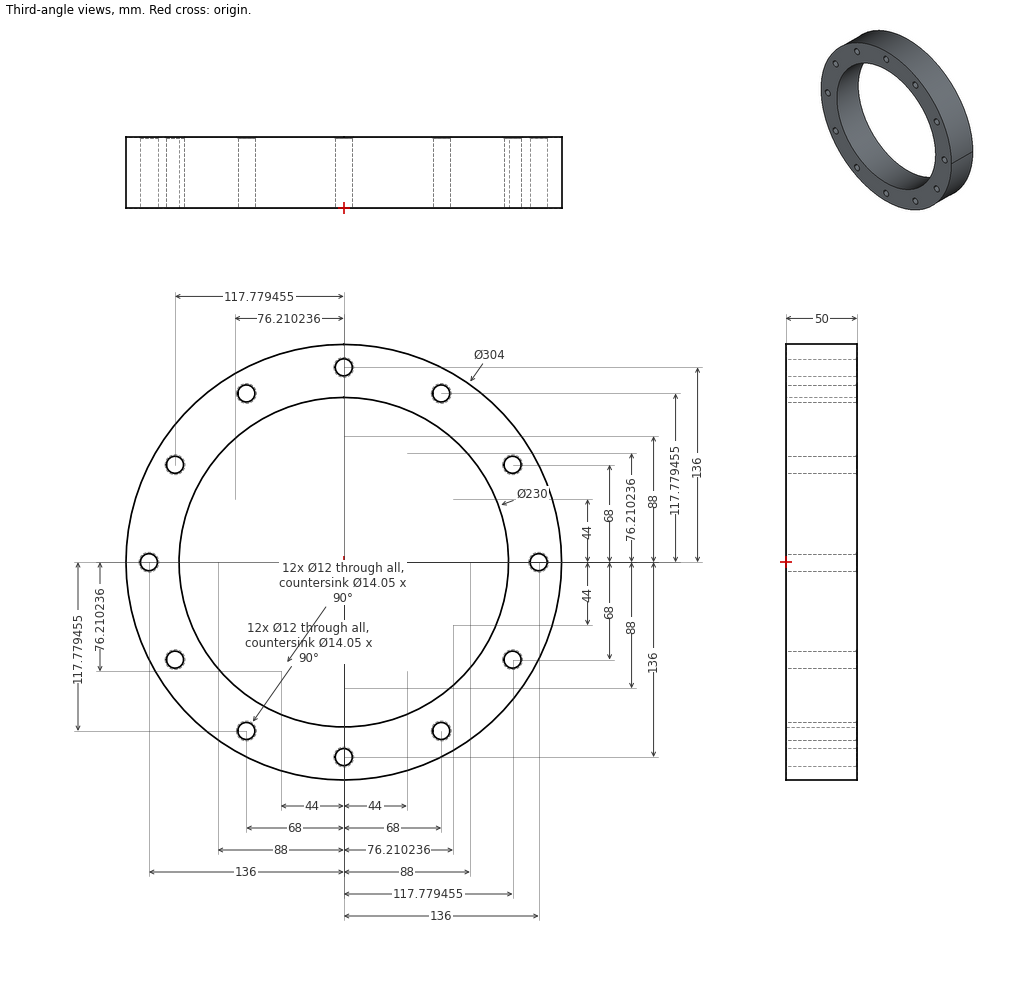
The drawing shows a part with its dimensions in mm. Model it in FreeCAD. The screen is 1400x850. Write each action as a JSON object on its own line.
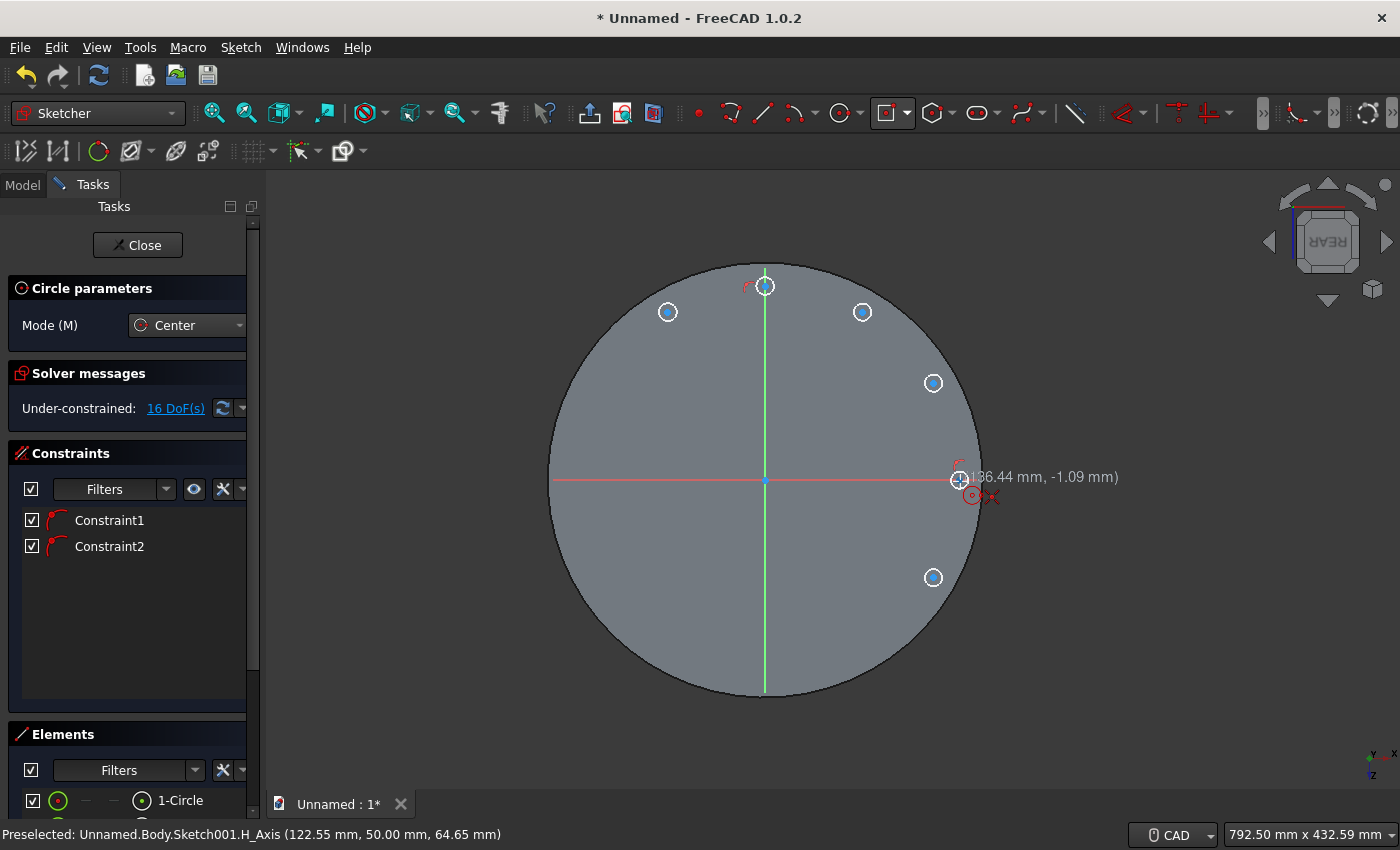
{"action": "scroll", "coordinate": [862, 649], "scroll_direction": "up", "scroll_amount": 5}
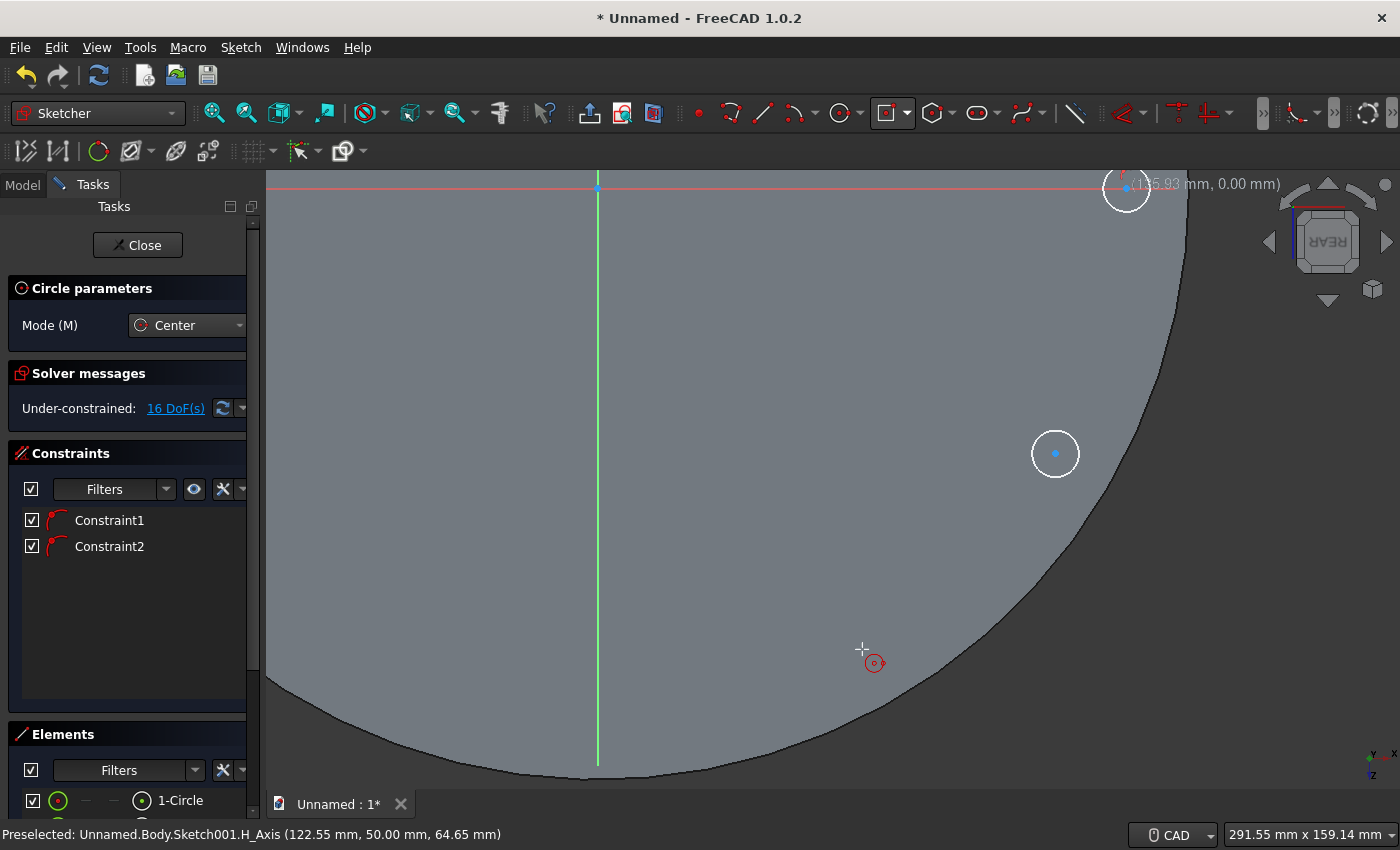
{"action": "left_click", "coordinate": [862, 647]}
{"action": "left_click", "coordinate": [879, 630]}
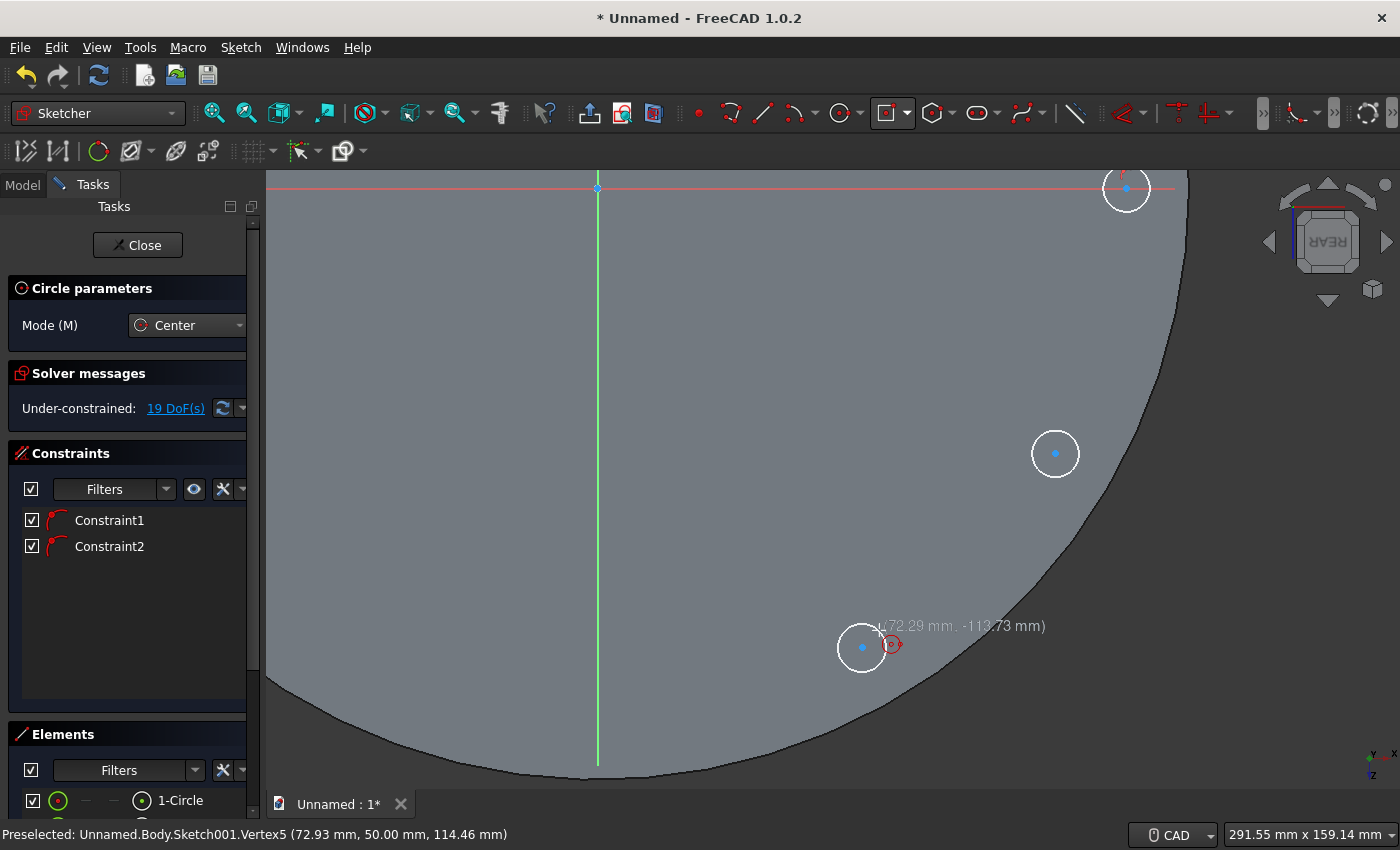
{"action": "left_click", "coordinate": [598, 718]}
{"action": "left_click", "coordinate": [614, 701]}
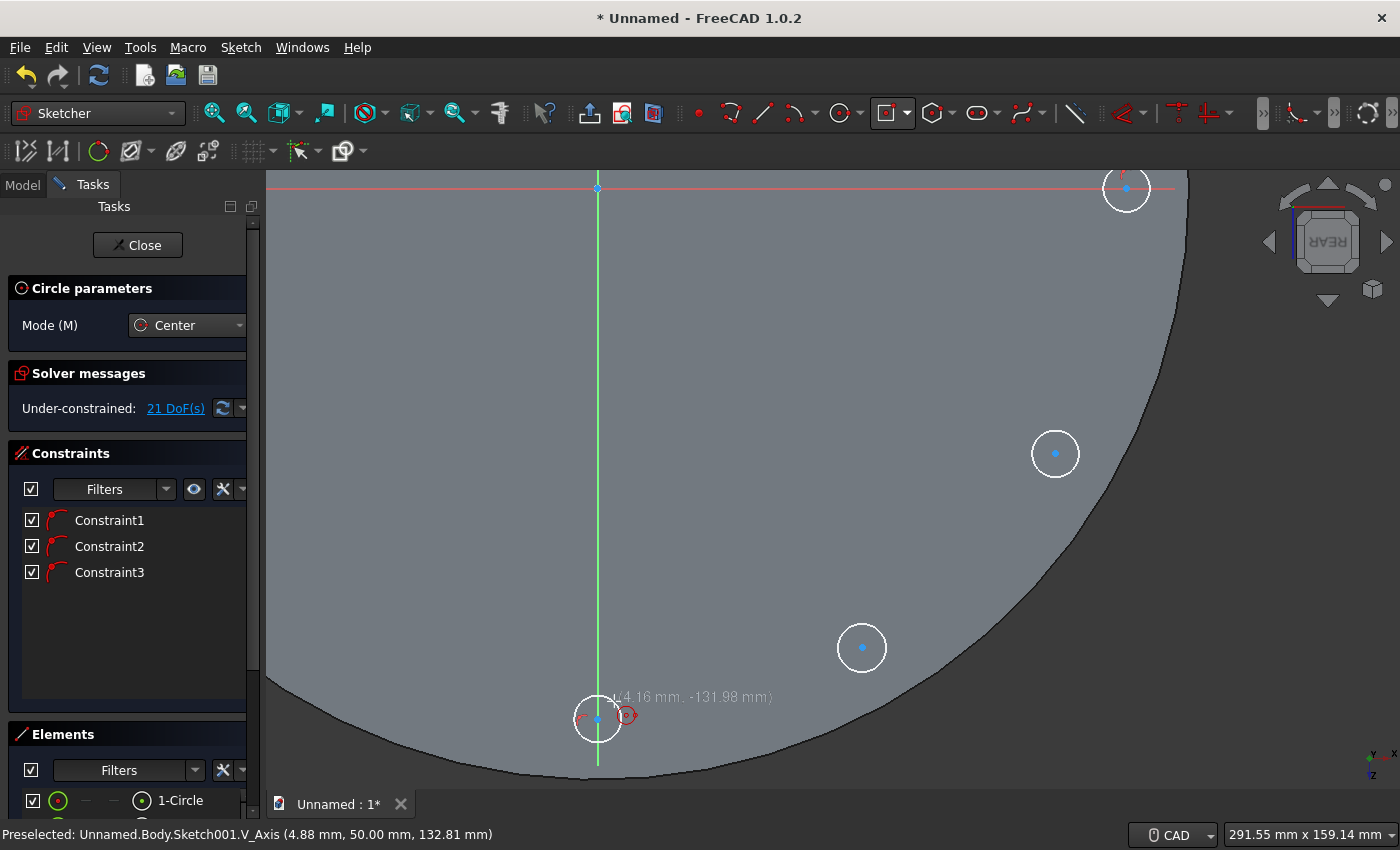
{"action": "left_click", "coordinate": [333, 647]}
{"action": "left_click", "coordinate": [350, 630]}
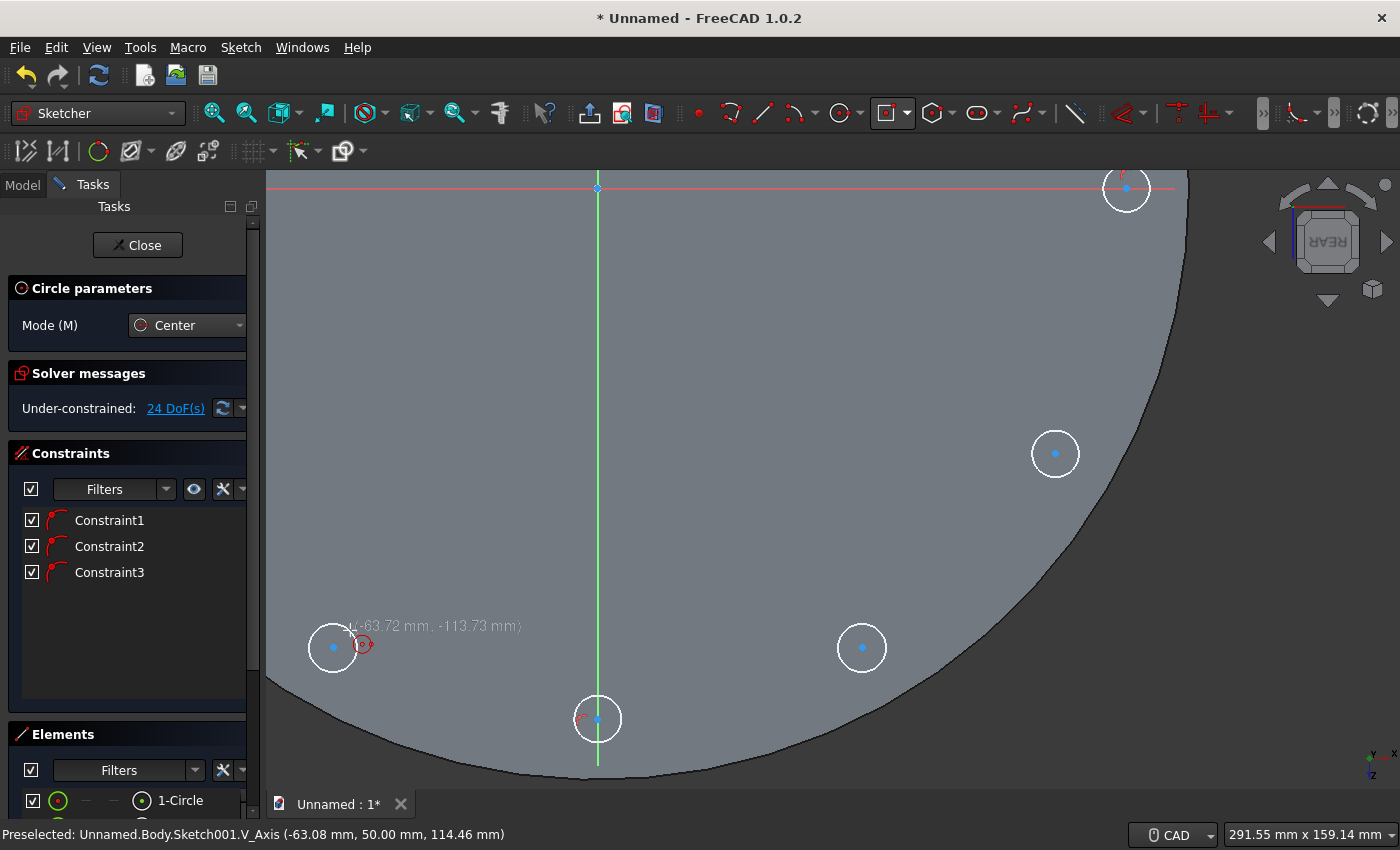
{"action": "scroll", "coordinate": [861, 649], "scroll_direction": "down", "scroll_amount": 5}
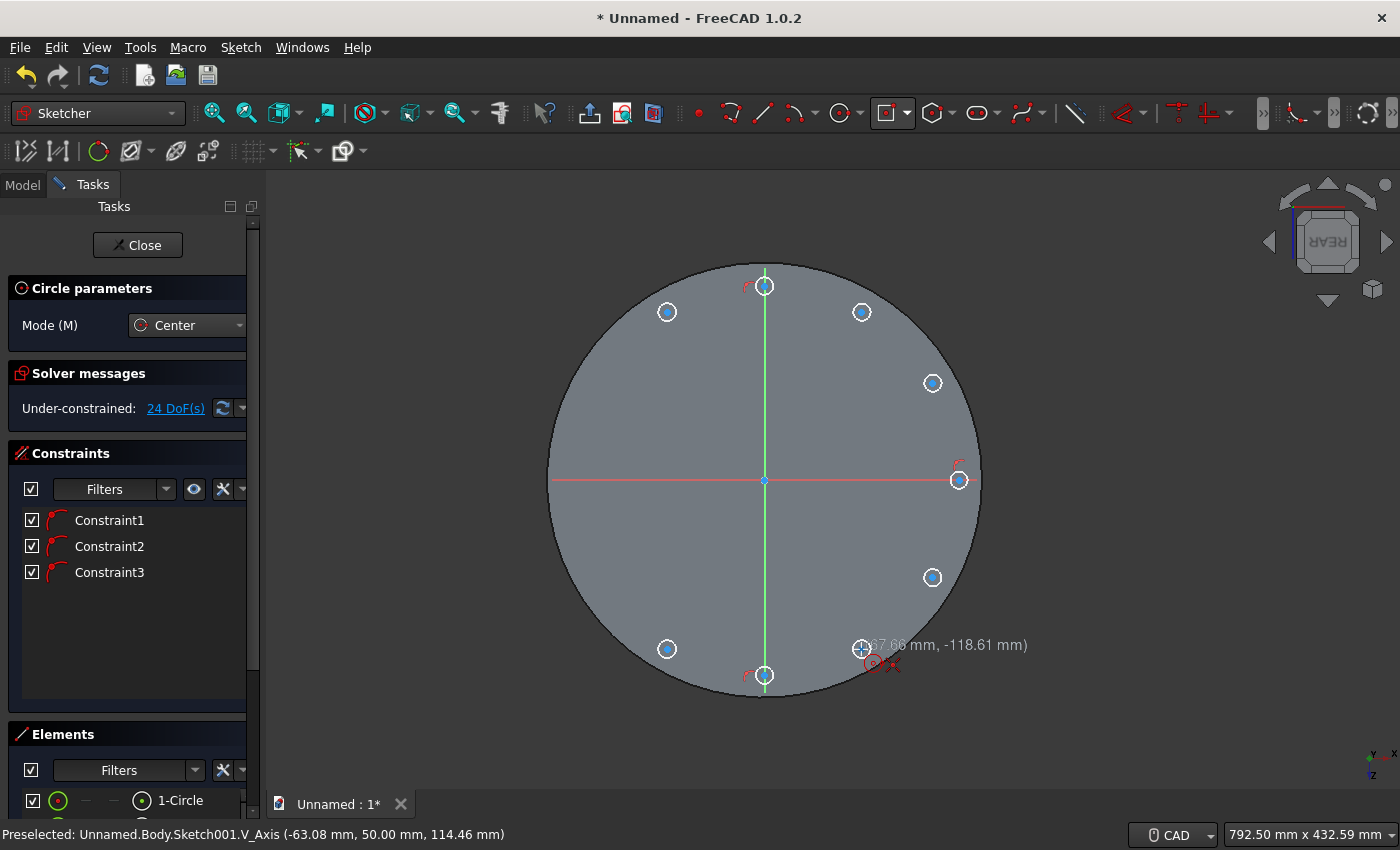
{"action": "scroll", "coordinate": [596, 577], "scroll_direction": "up", "scroll_amount": 5}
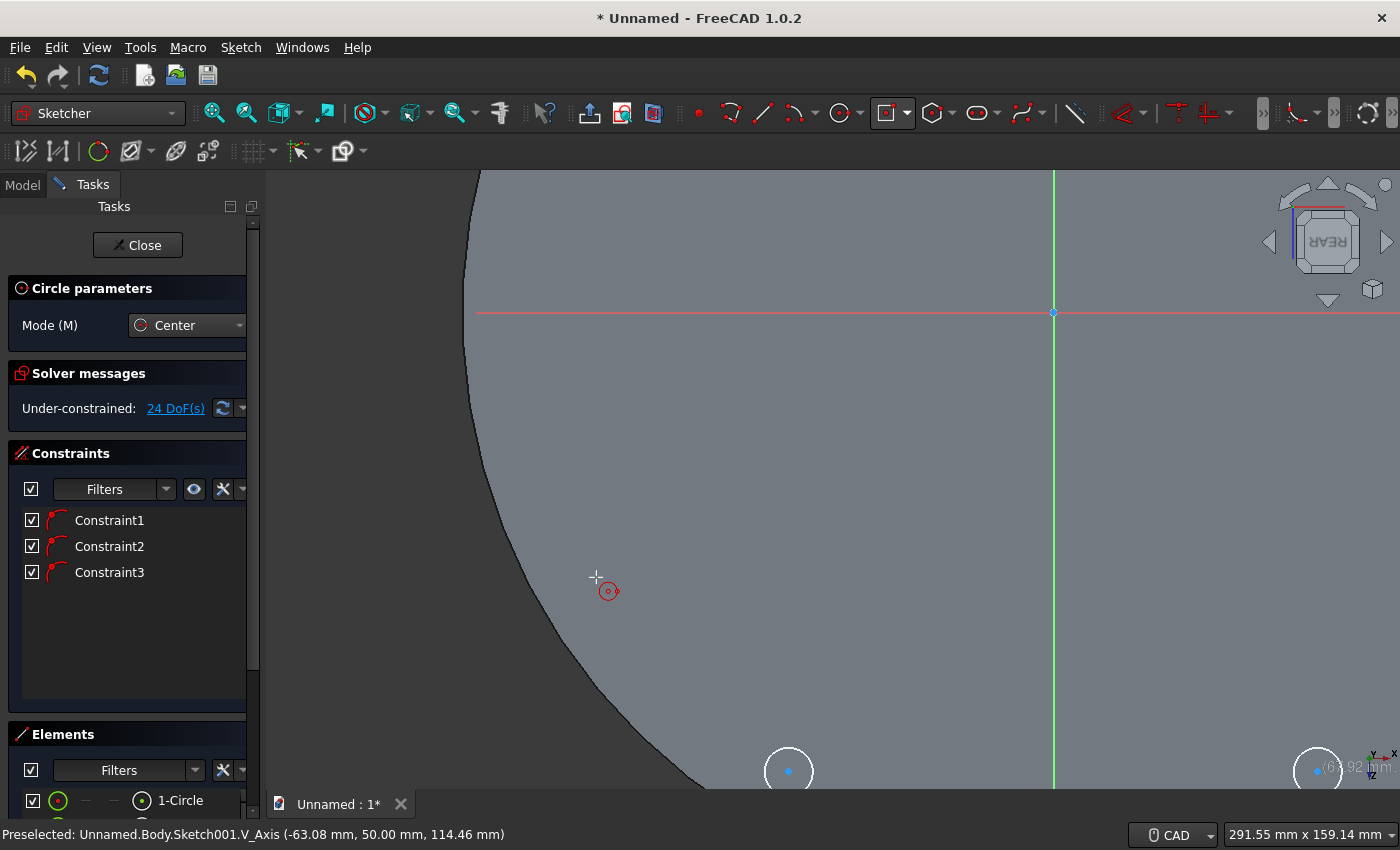
{"action": "left_click", "coordinate": [595, 577]}
{"action": "left_click", "coordinate": [612, 561]}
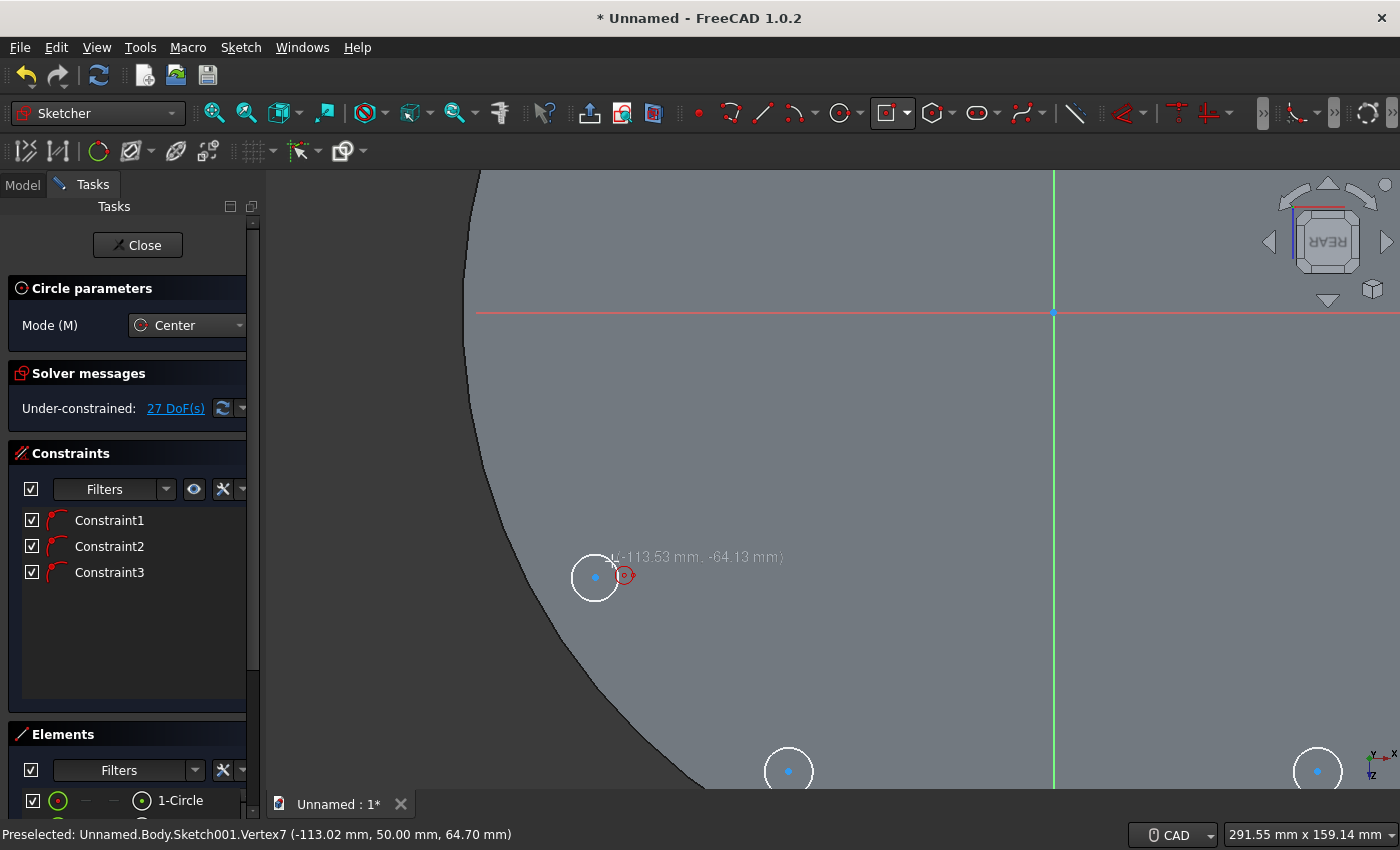
{"action": "left_click", "coordinate": [525, 313]}
{"action": "left_click", "coordinate": [541, 296]}